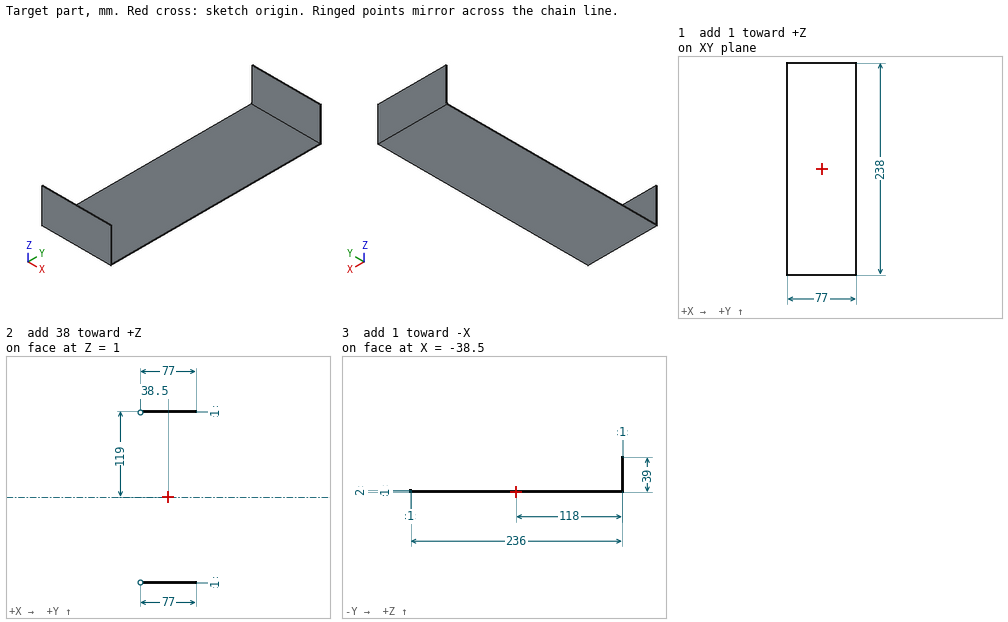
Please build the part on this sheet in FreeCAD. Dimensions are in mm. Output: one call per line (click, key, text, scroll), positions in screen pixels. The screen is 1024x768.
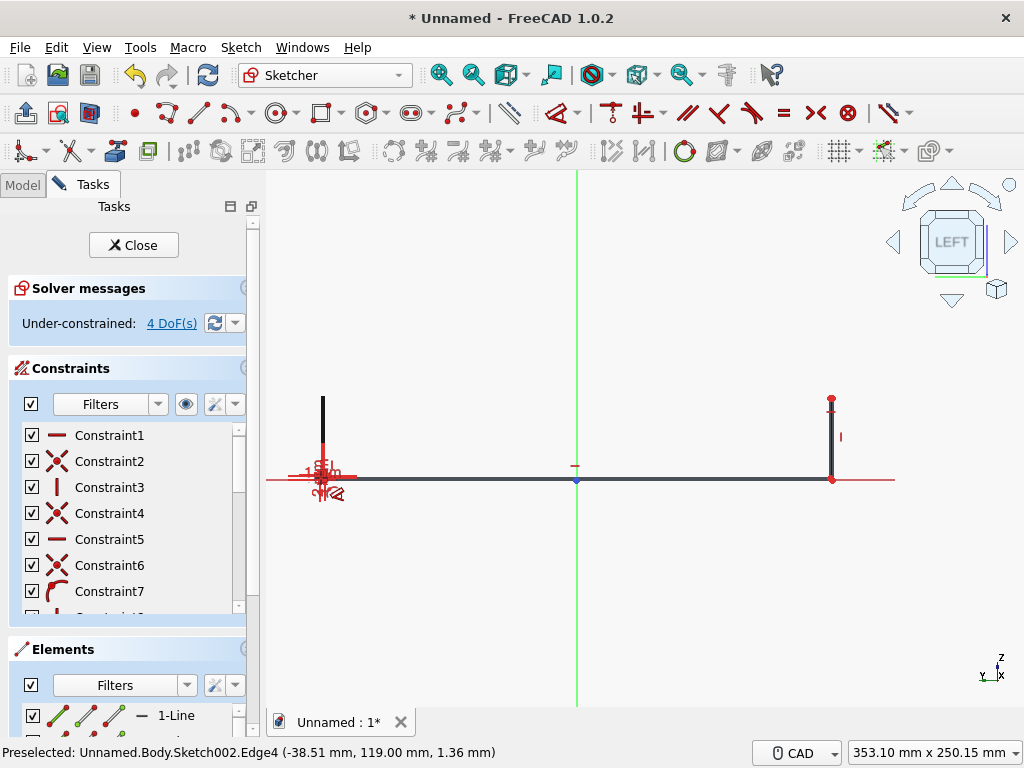
scroll(832, 398, up, 15)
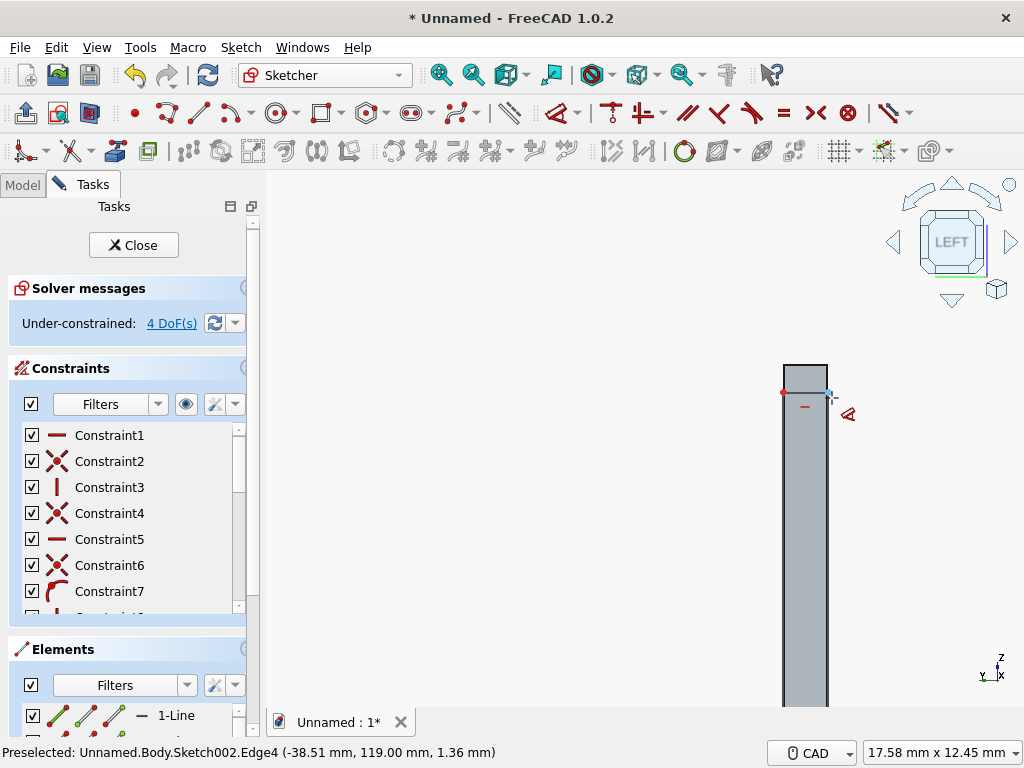
click(815, 393)
click(806, 359)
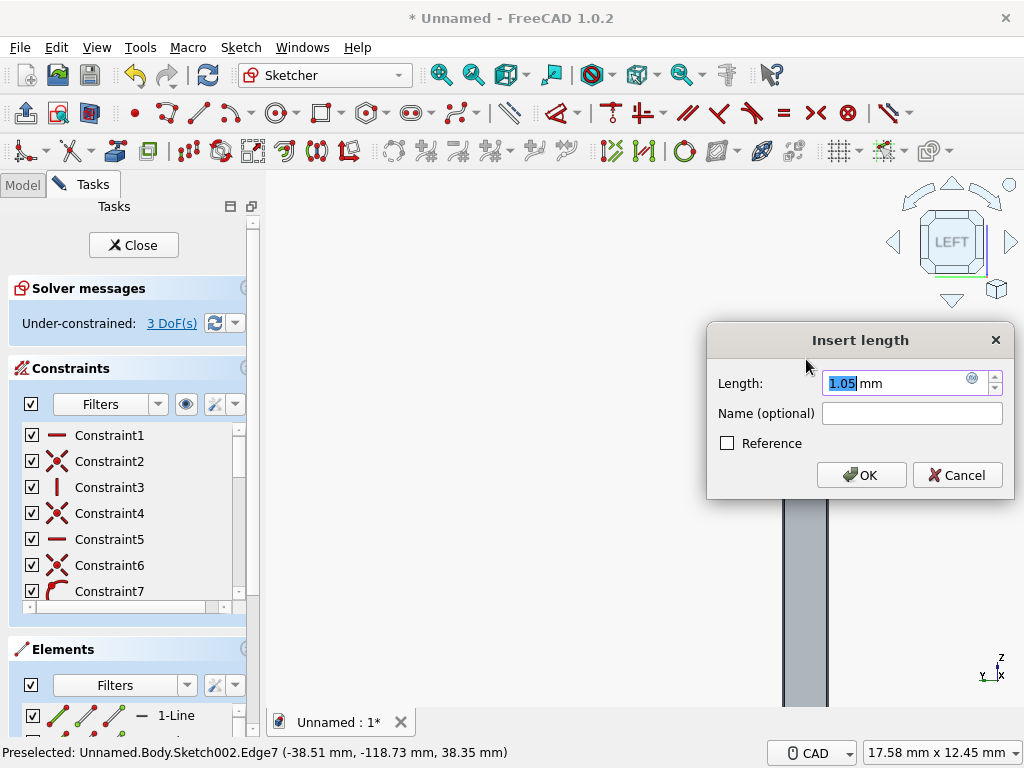
text(1)
key(Return)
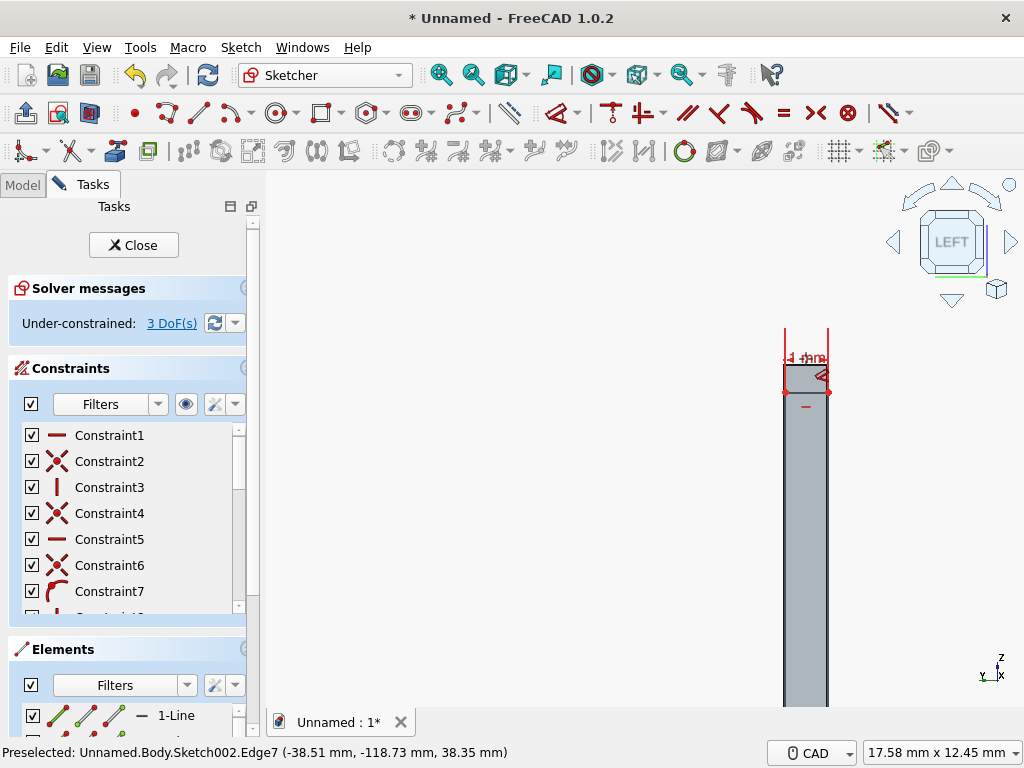
scroll(832, 398, down, 15)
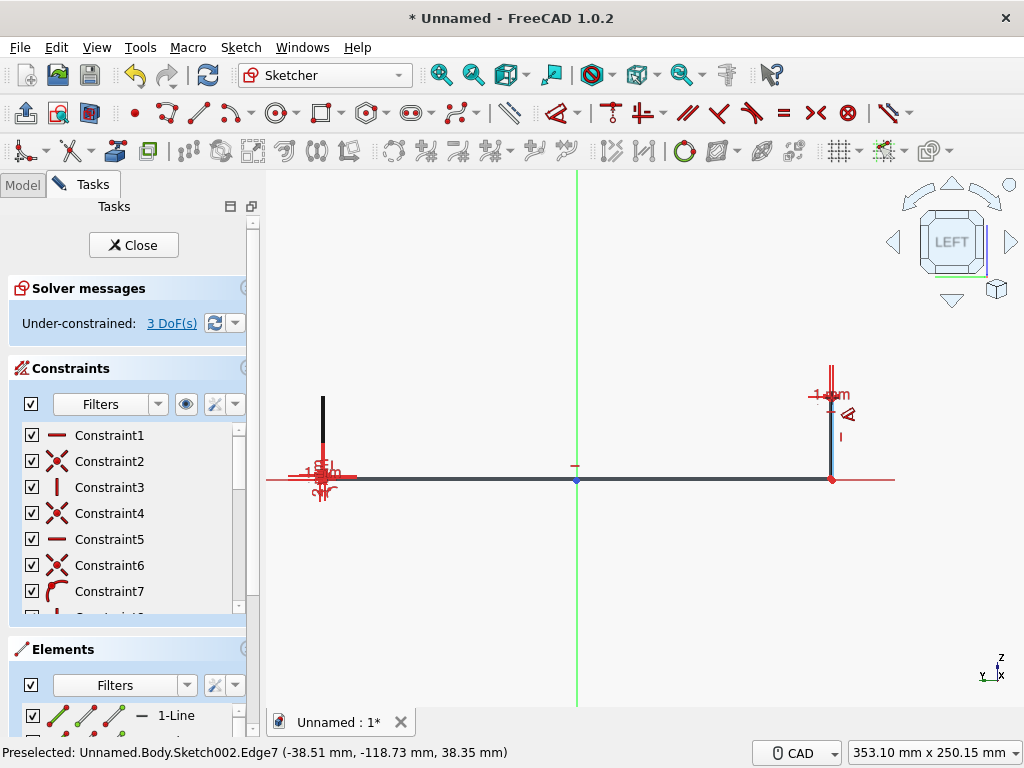
scroll(833, 456, up, 10)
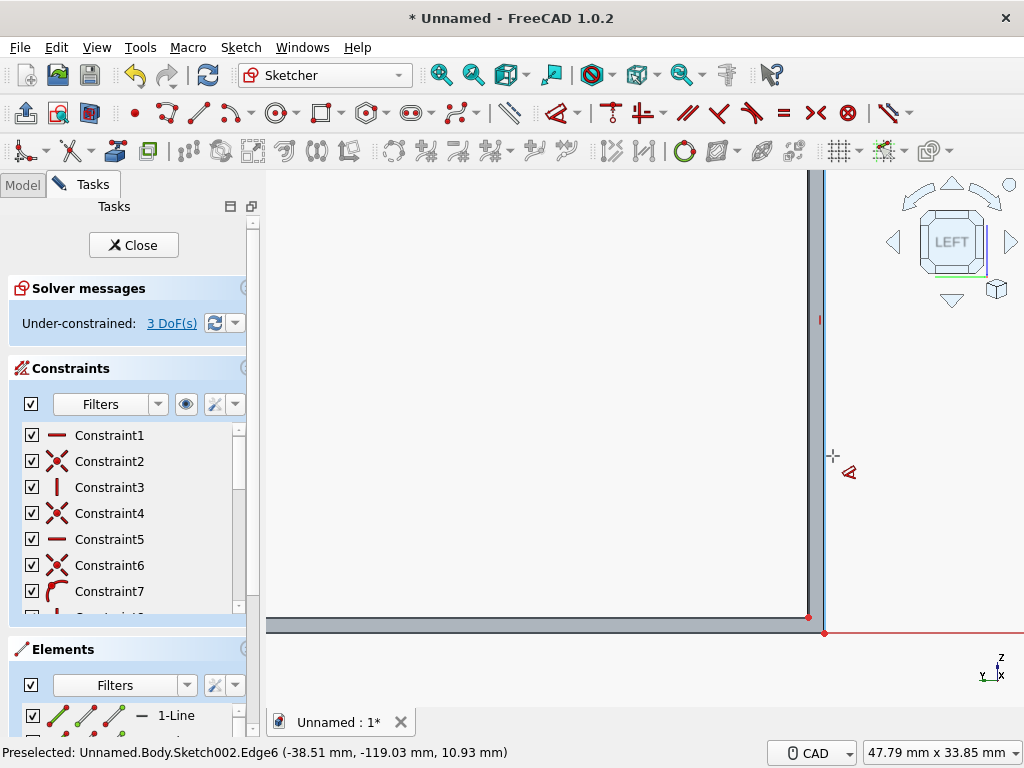
click(825, 451)
click(859, 416)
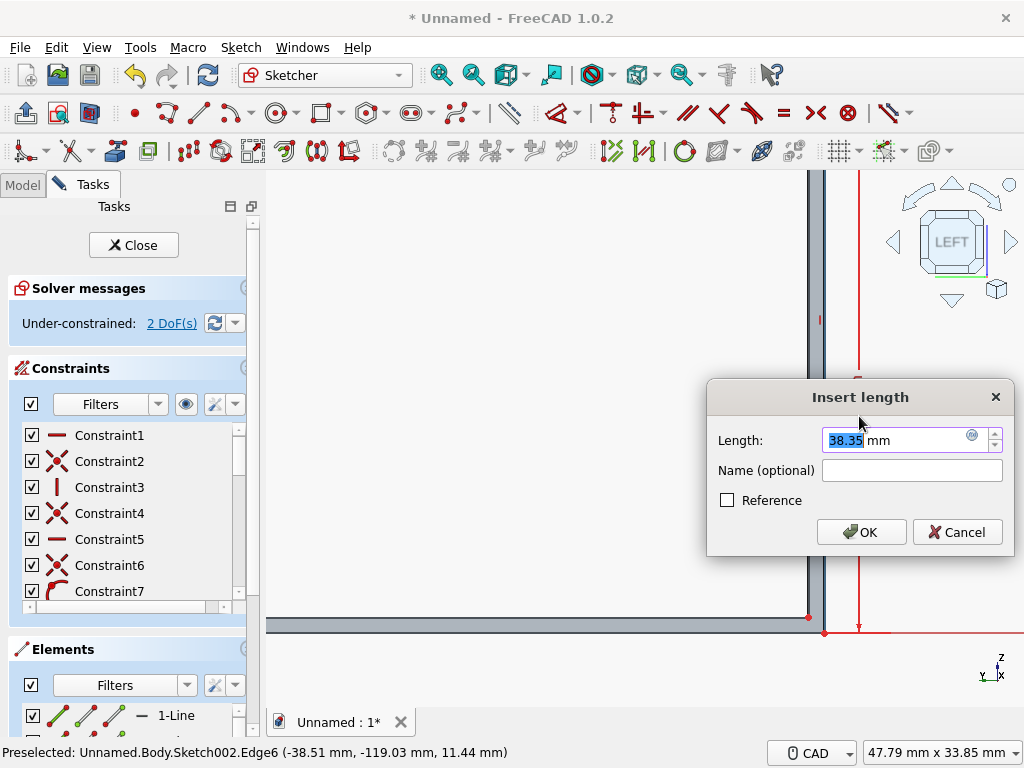
text(39)
key(Return)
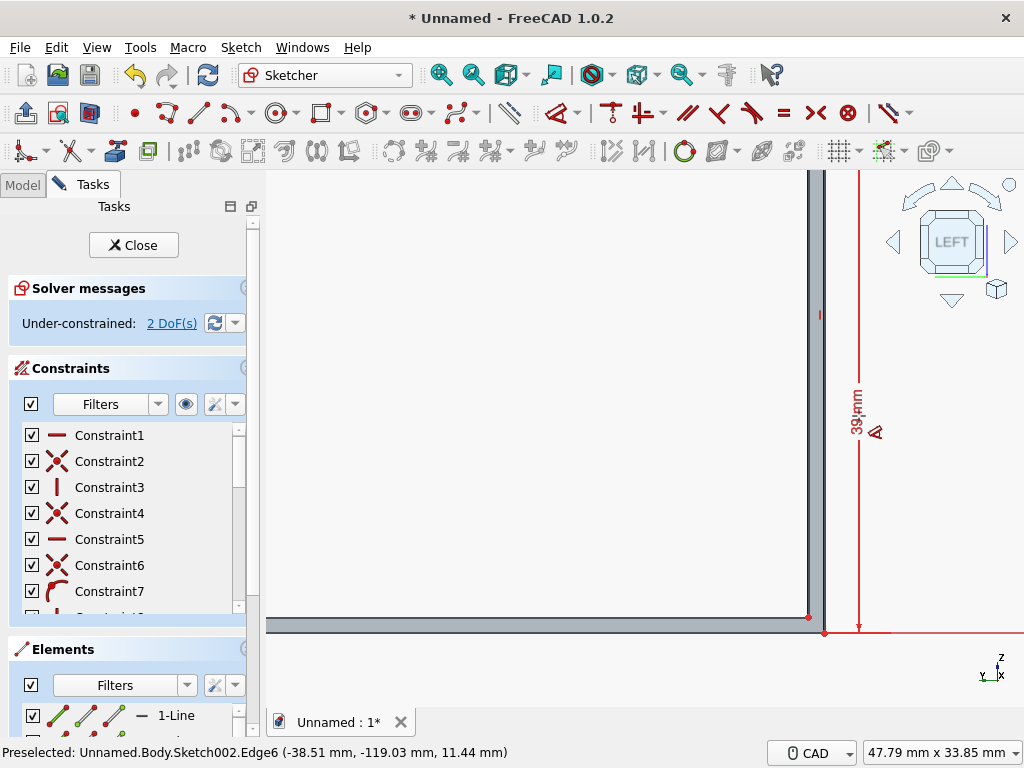
scroll(781, 453, down, 11)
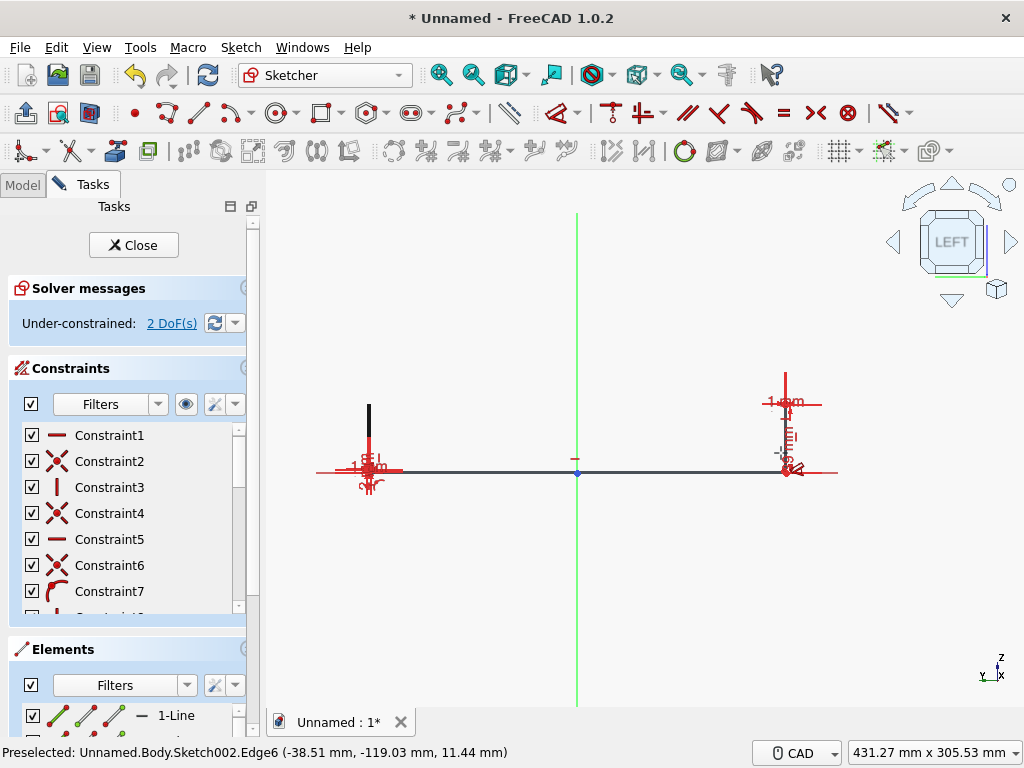
scroll(660, 472, up, 11)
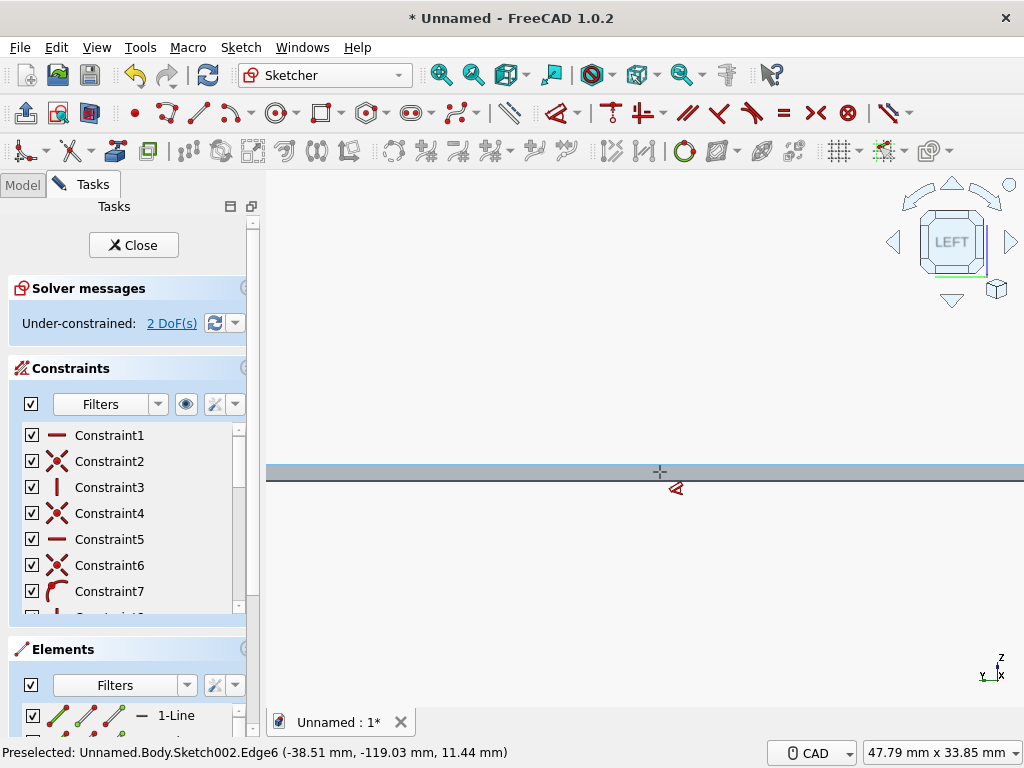
click(658, 465)
click(576, 499)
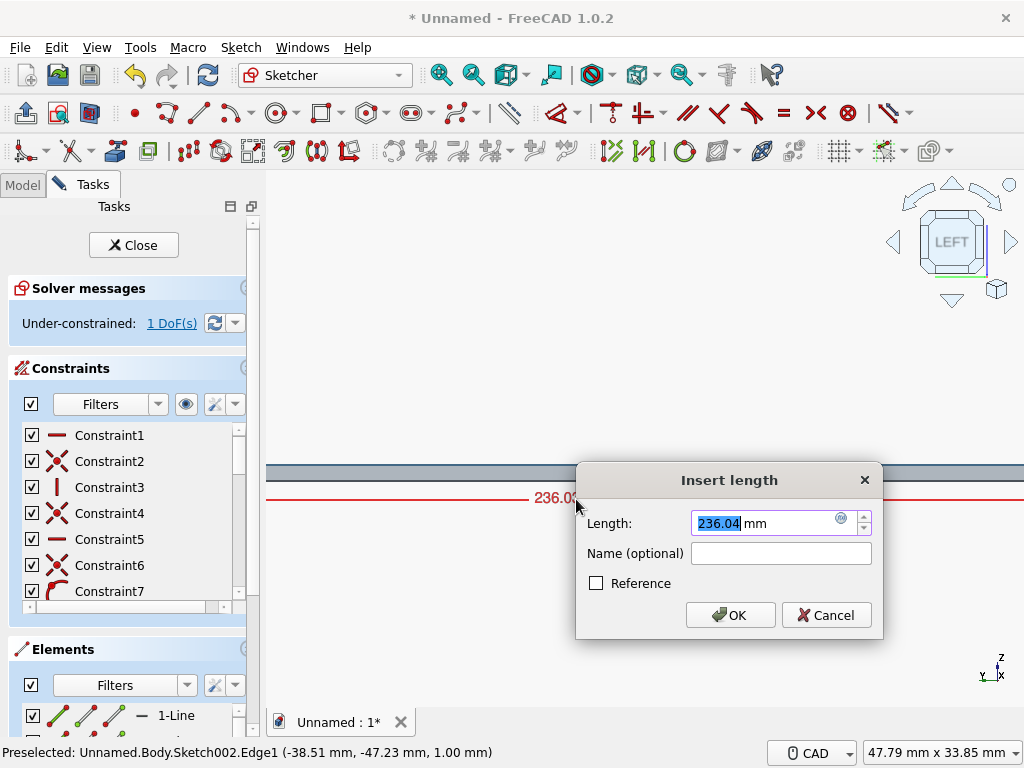
text(236)
key(Return)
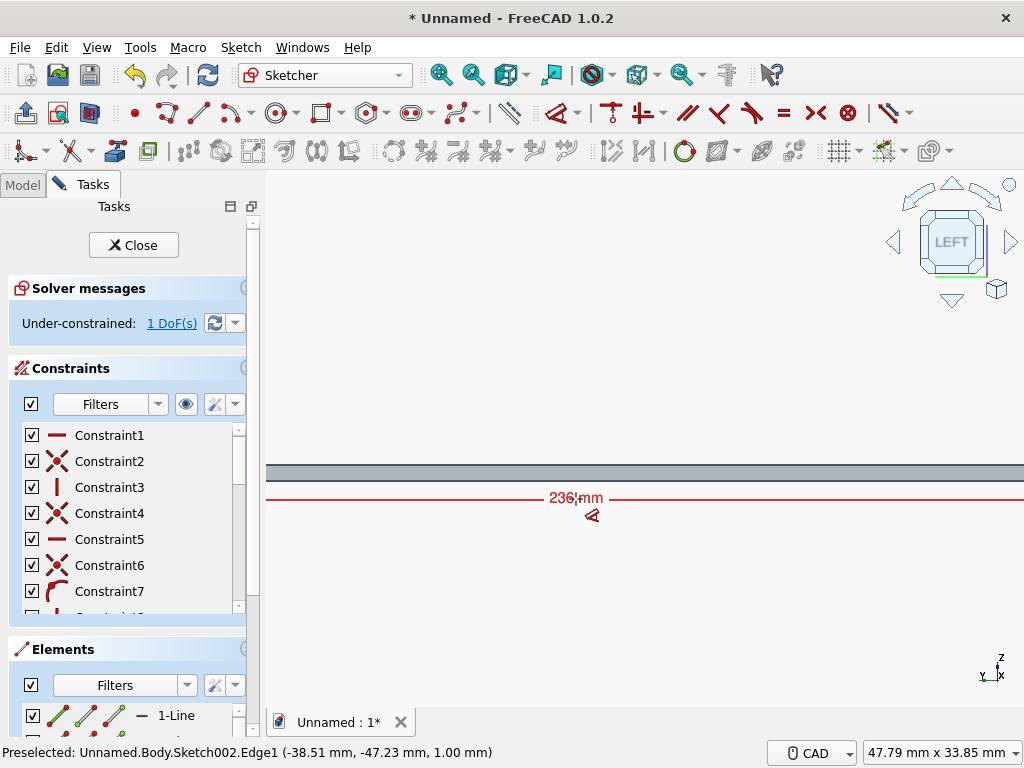
scroll(660, 472, down, 11)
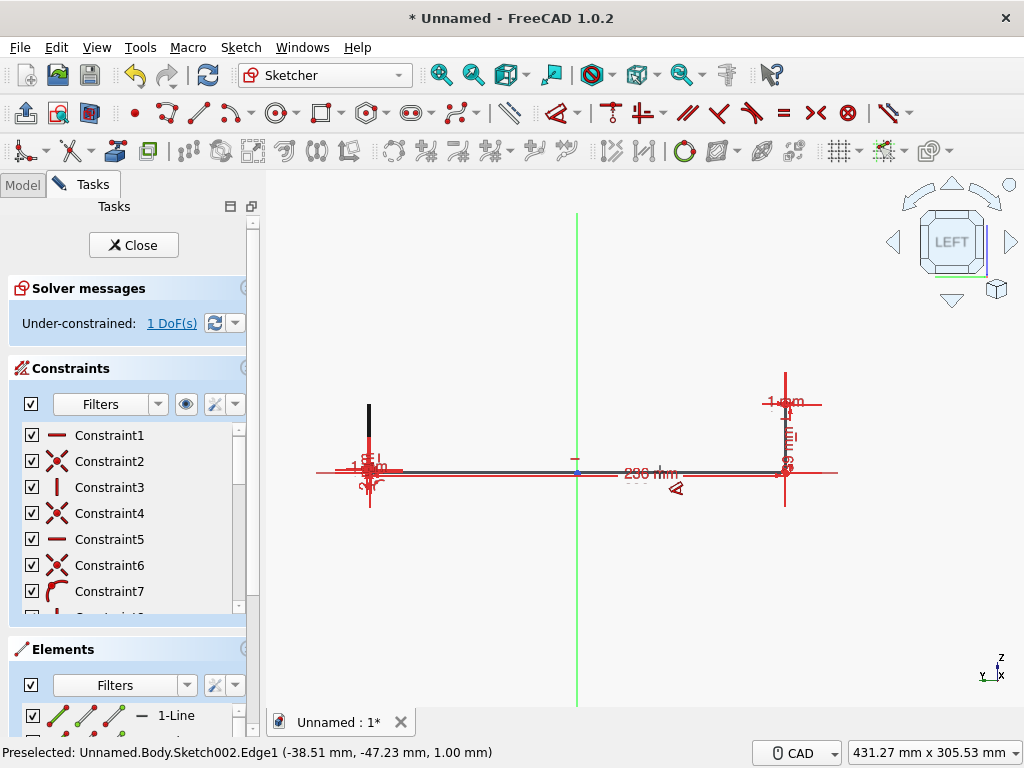
scroll(785, 472, up, 8)